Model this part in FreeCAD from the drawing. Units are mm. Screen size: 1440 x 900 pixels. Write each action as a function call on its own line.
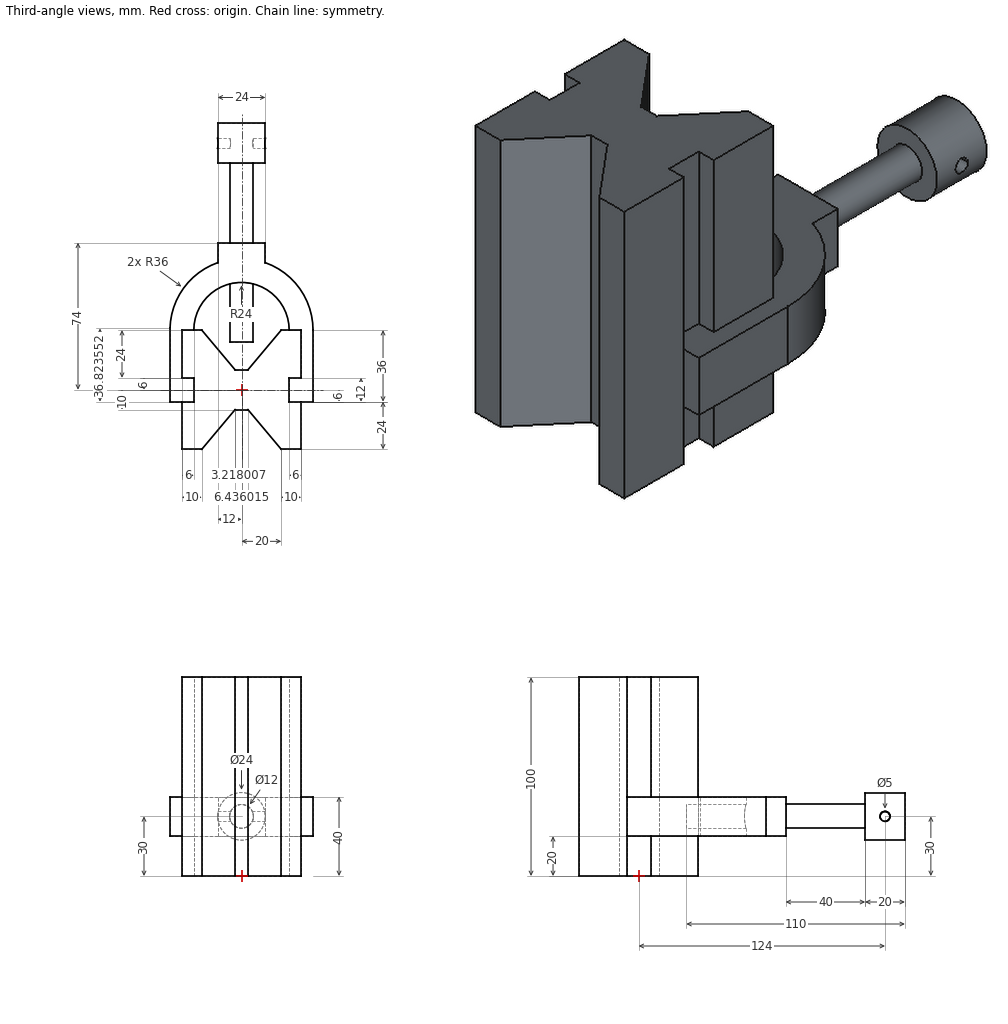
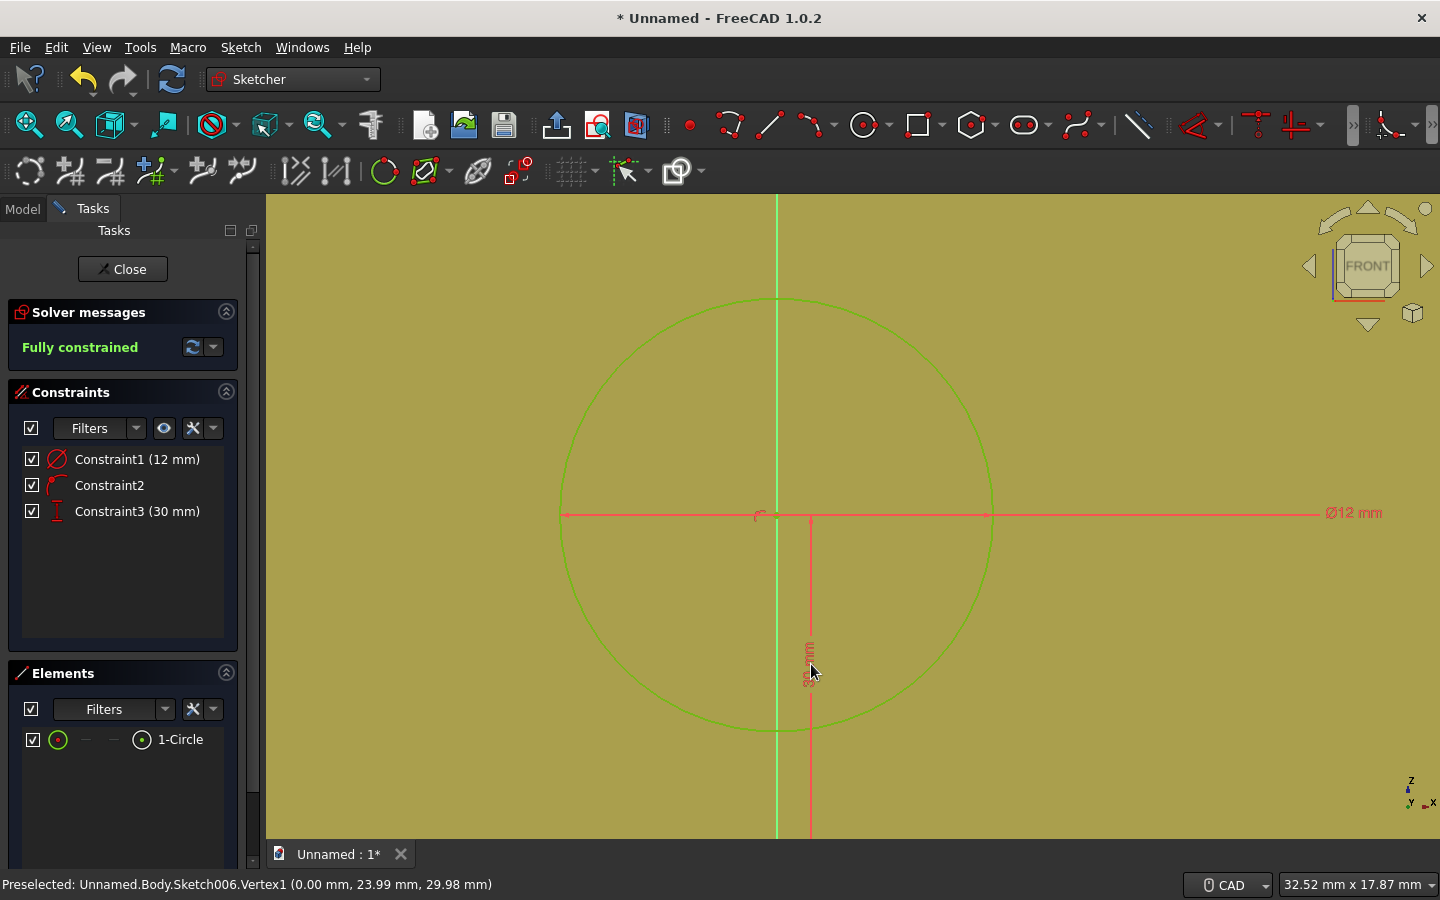
click(123, 269)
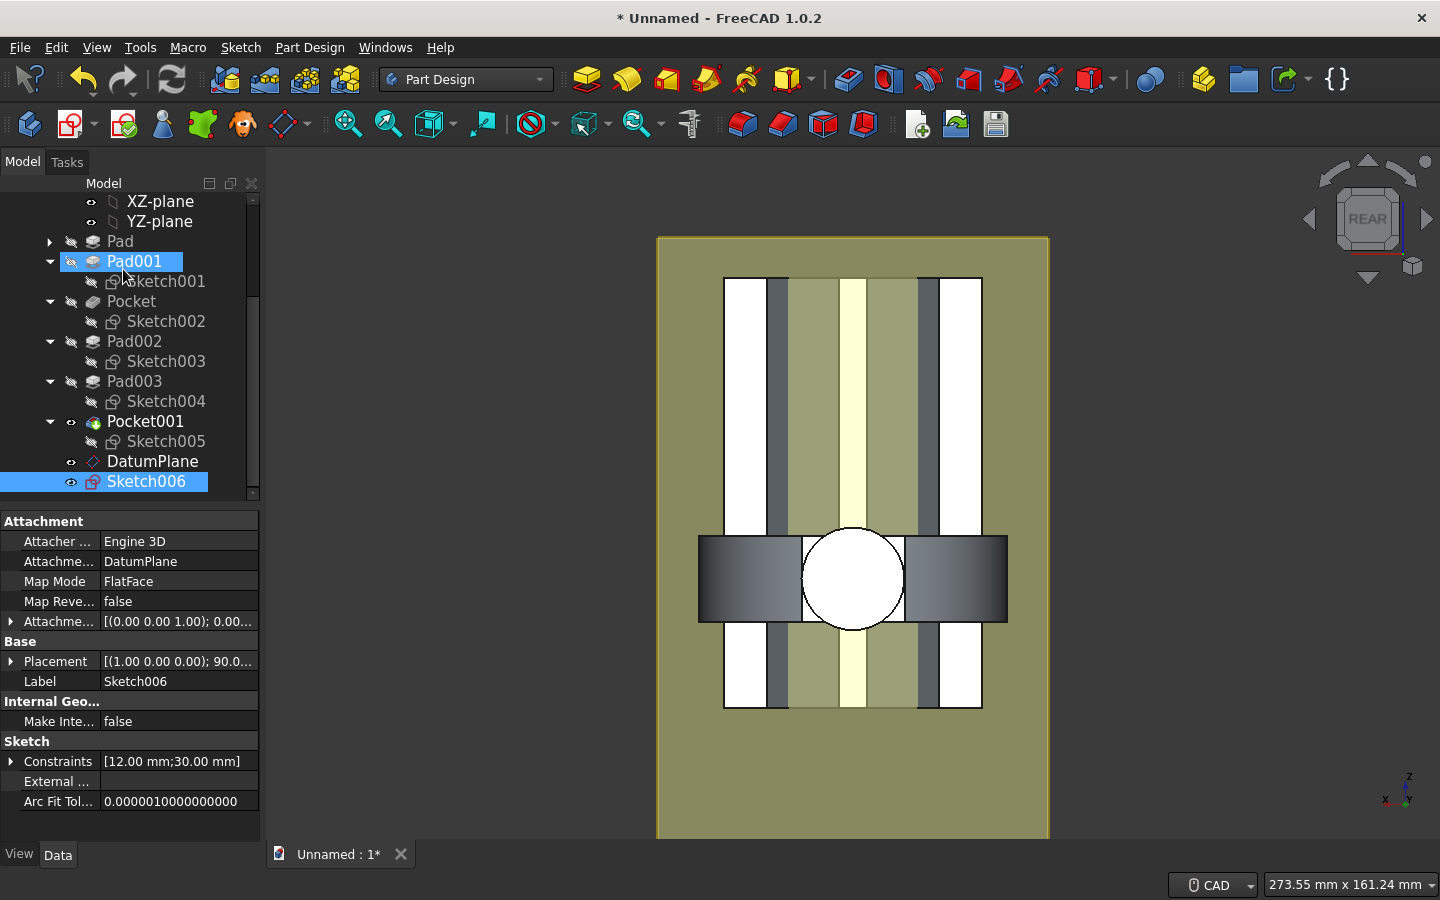
click(588, 80)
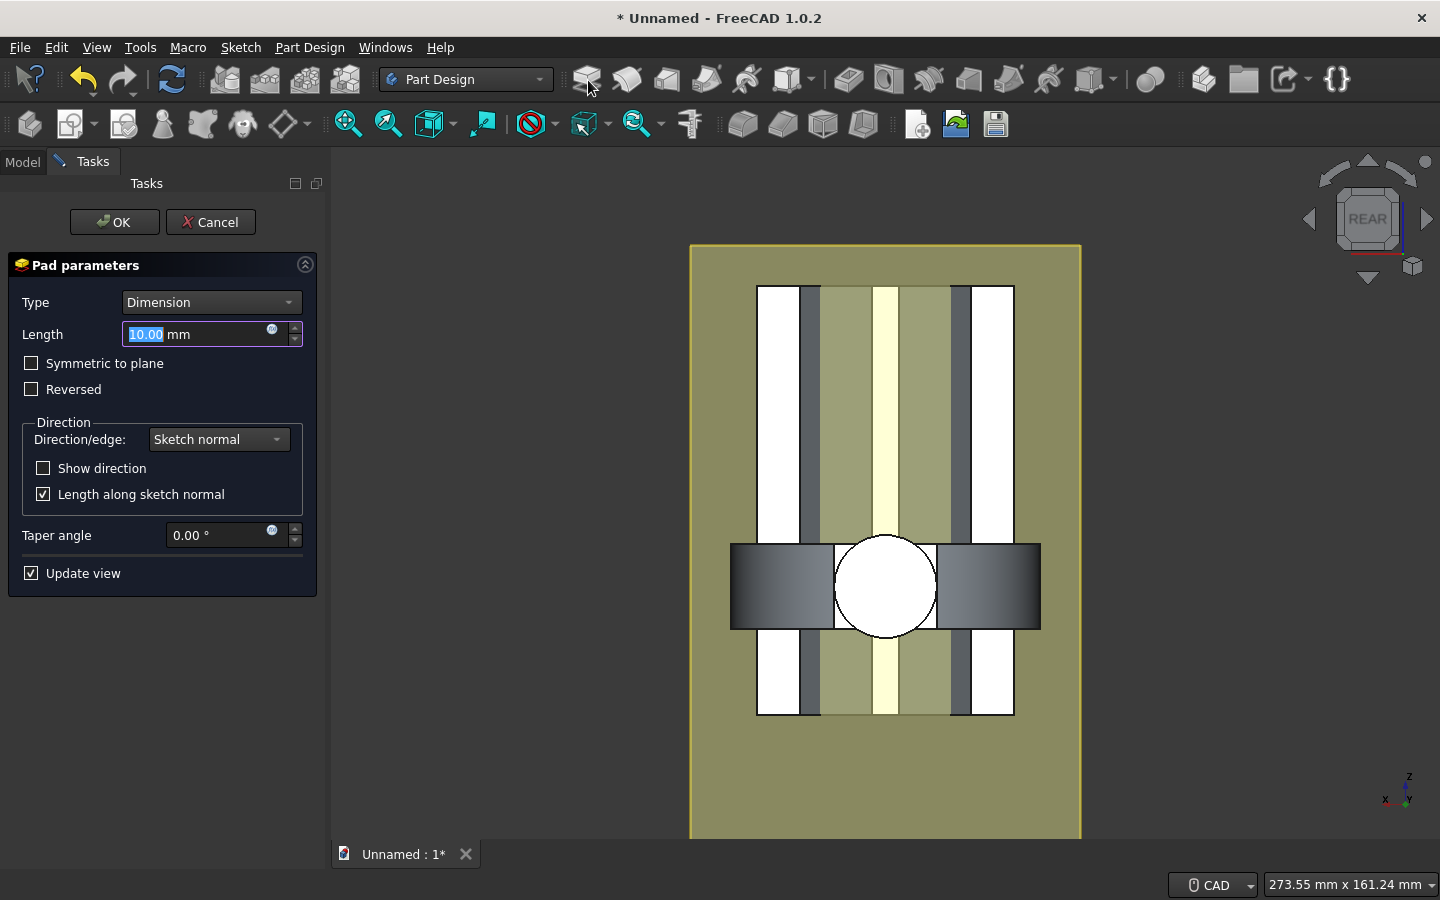
text(110)
key(Tab)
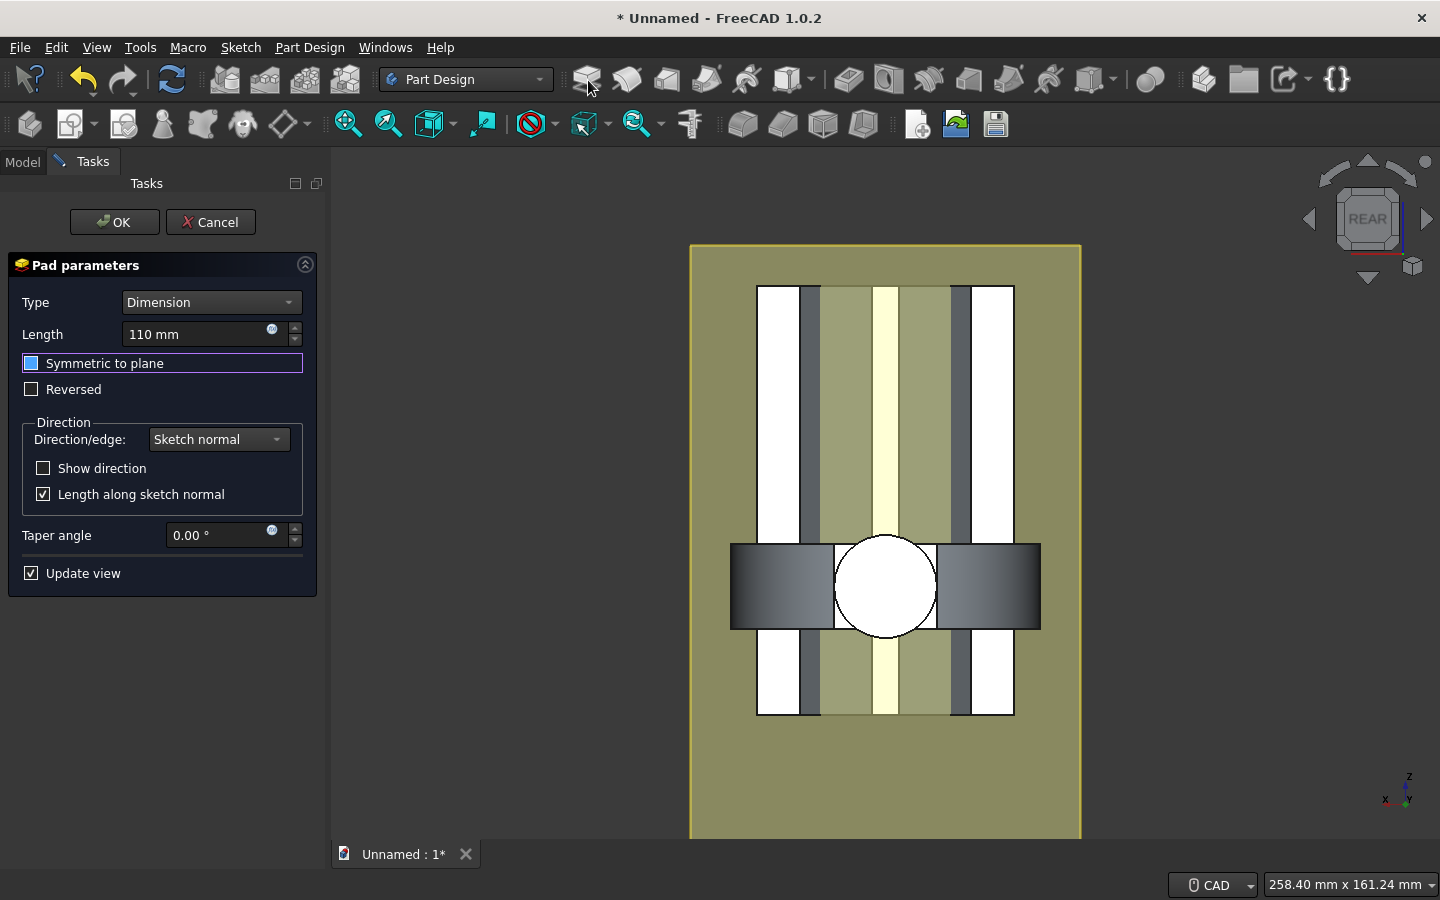
click(30, 389)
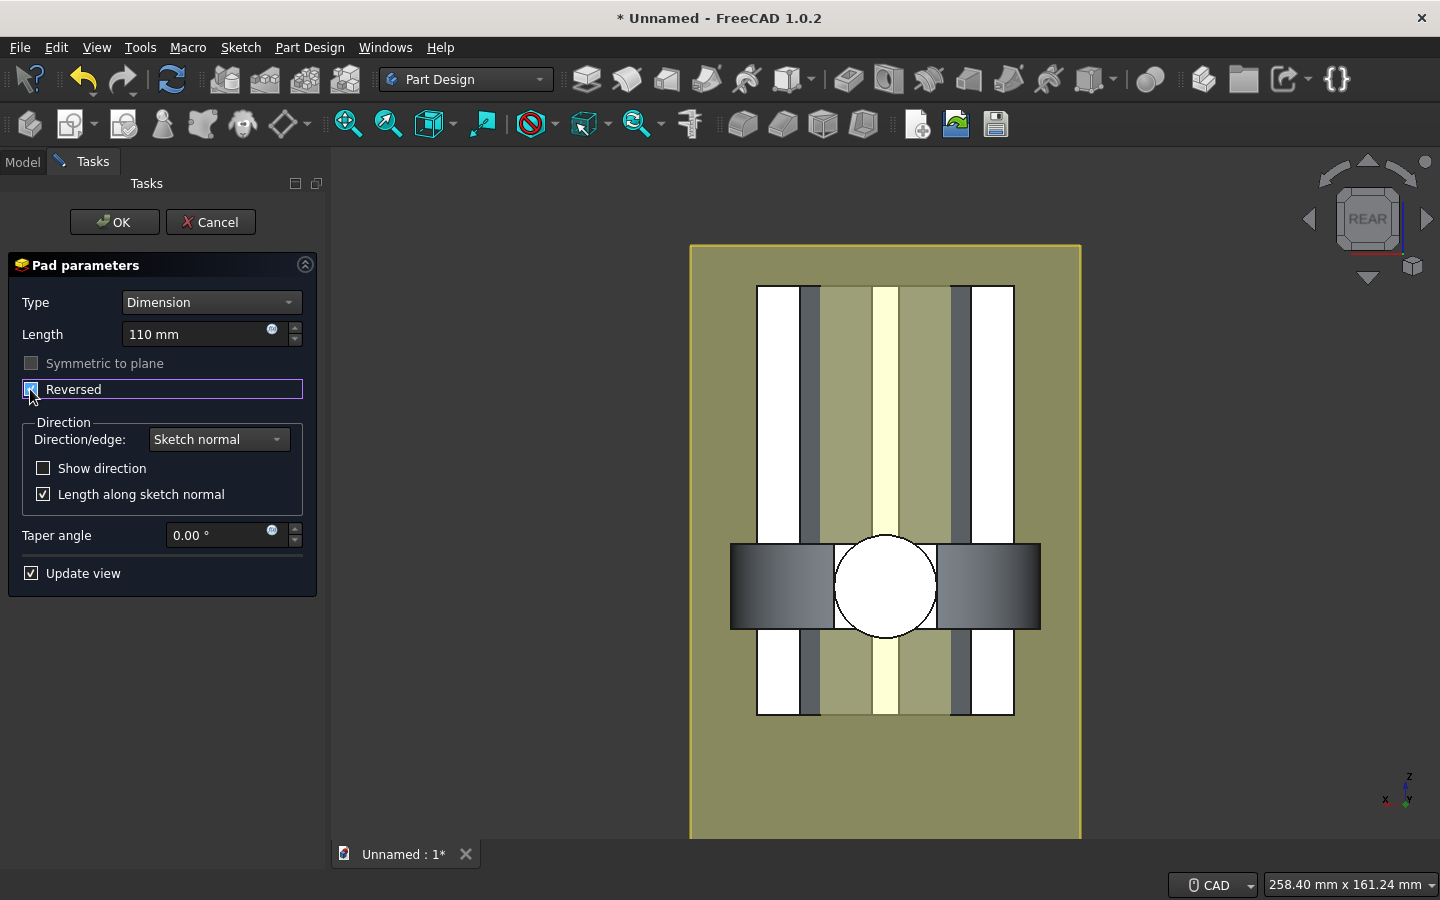
click(115, 222)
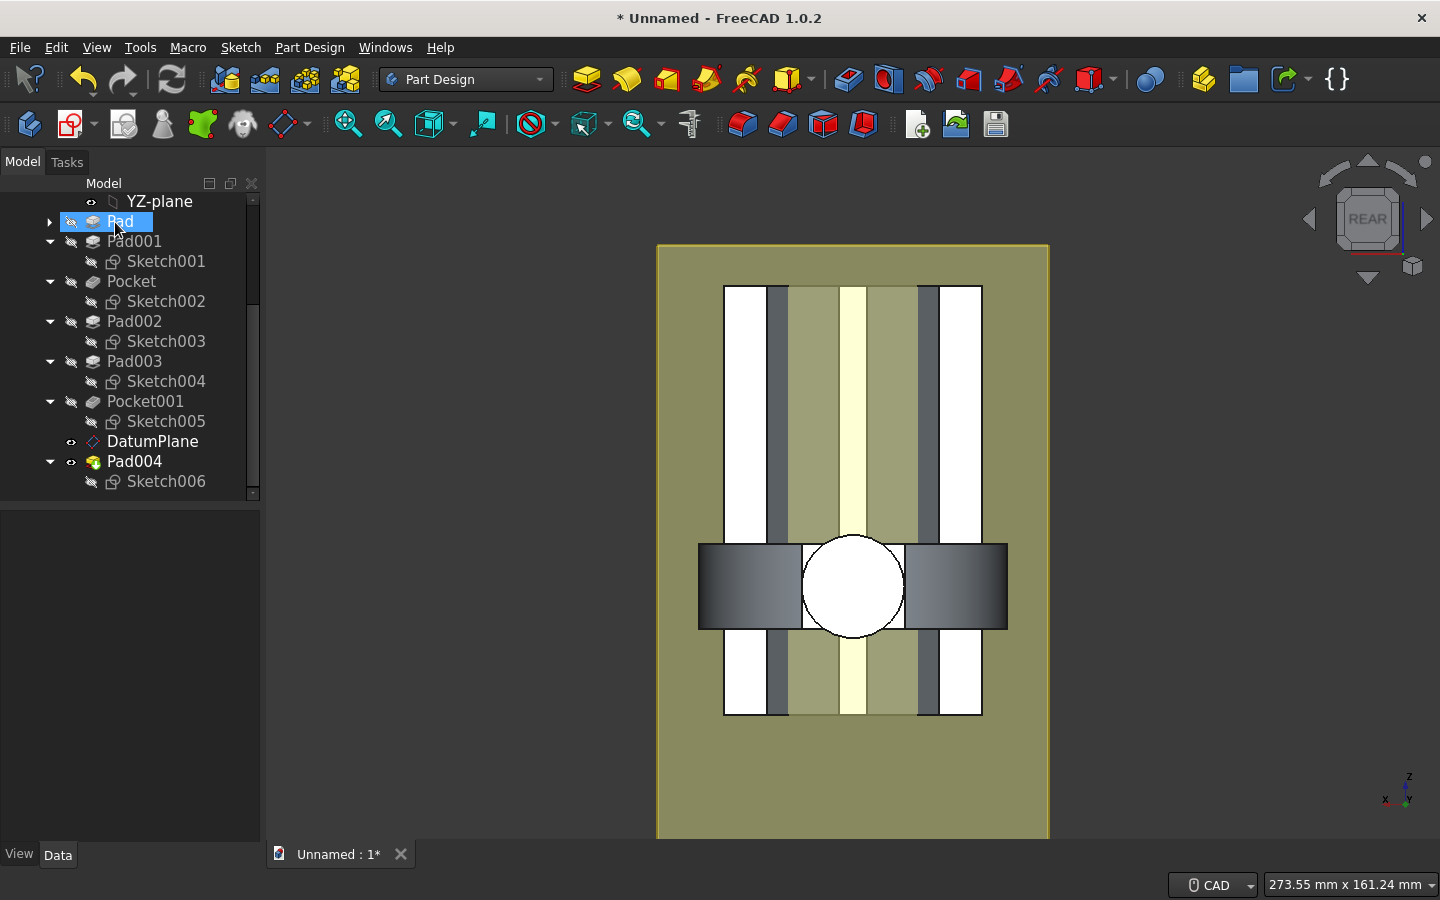
click(116, 442)
key(space)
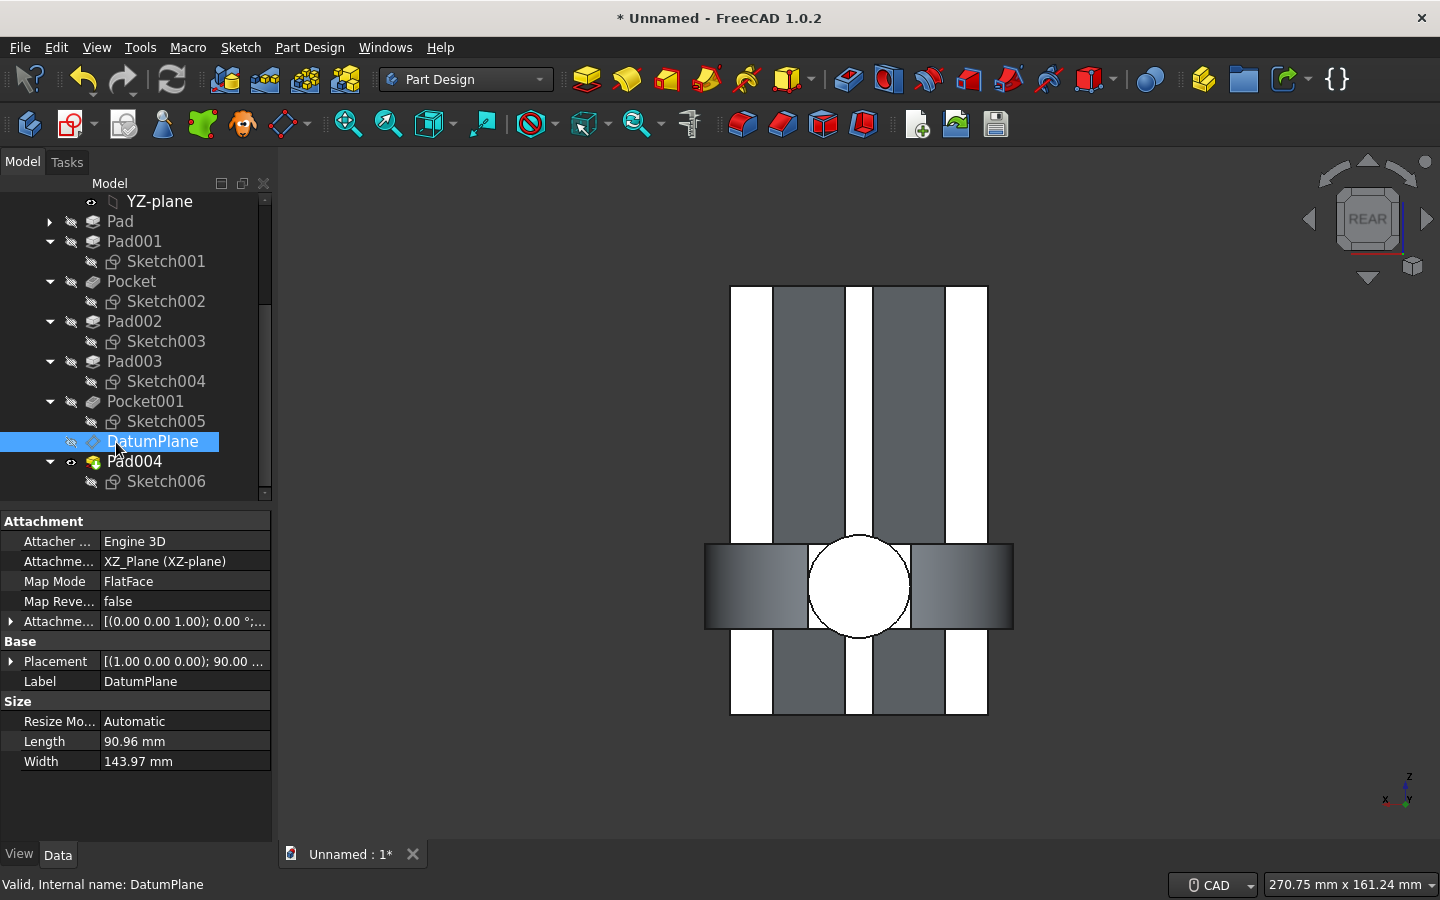
key(0)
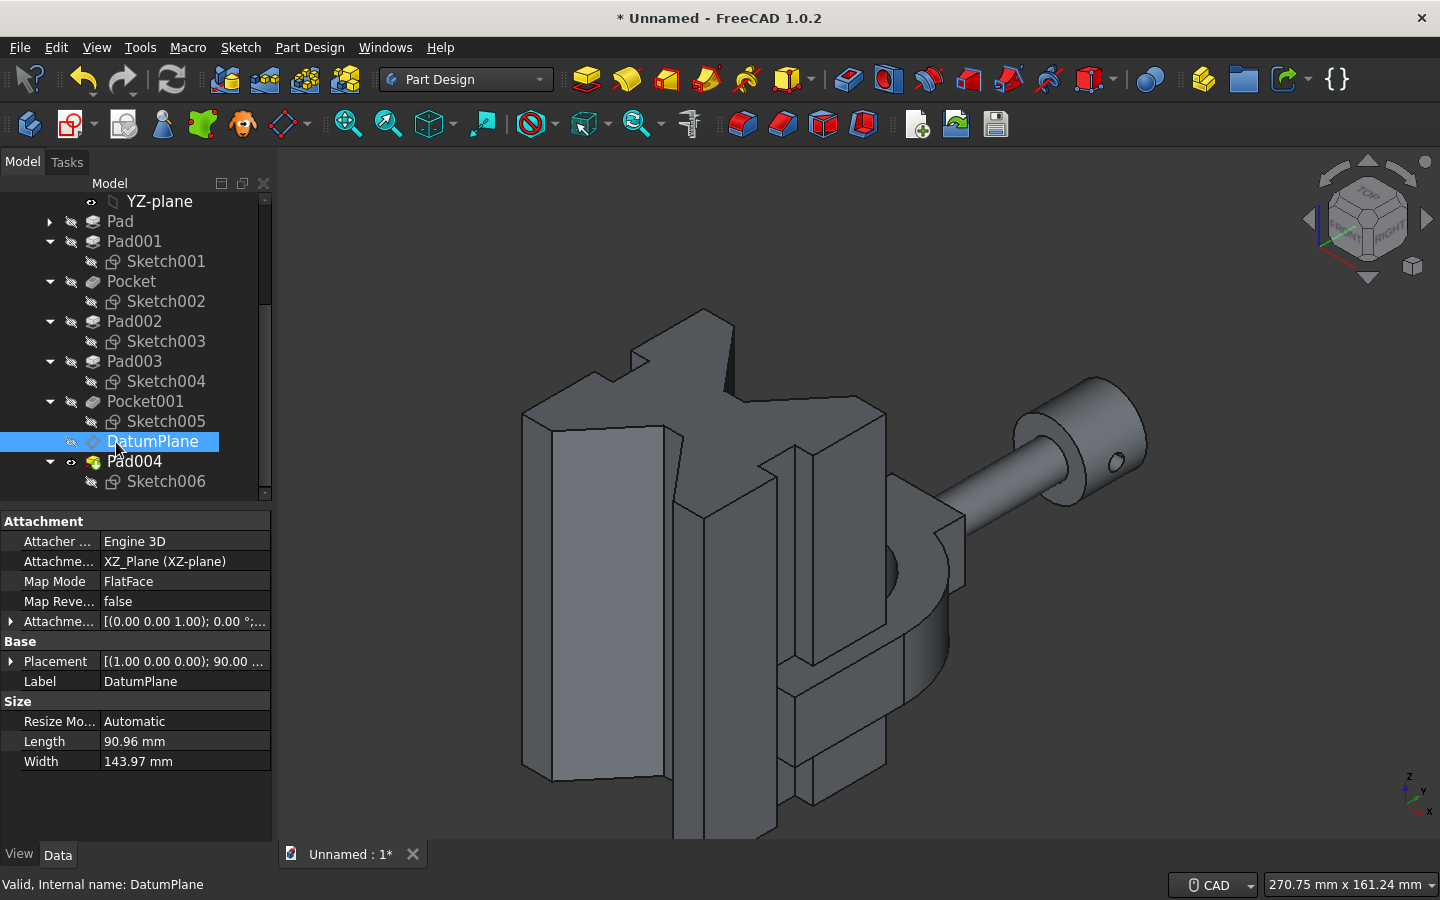
key(v)
key(f)